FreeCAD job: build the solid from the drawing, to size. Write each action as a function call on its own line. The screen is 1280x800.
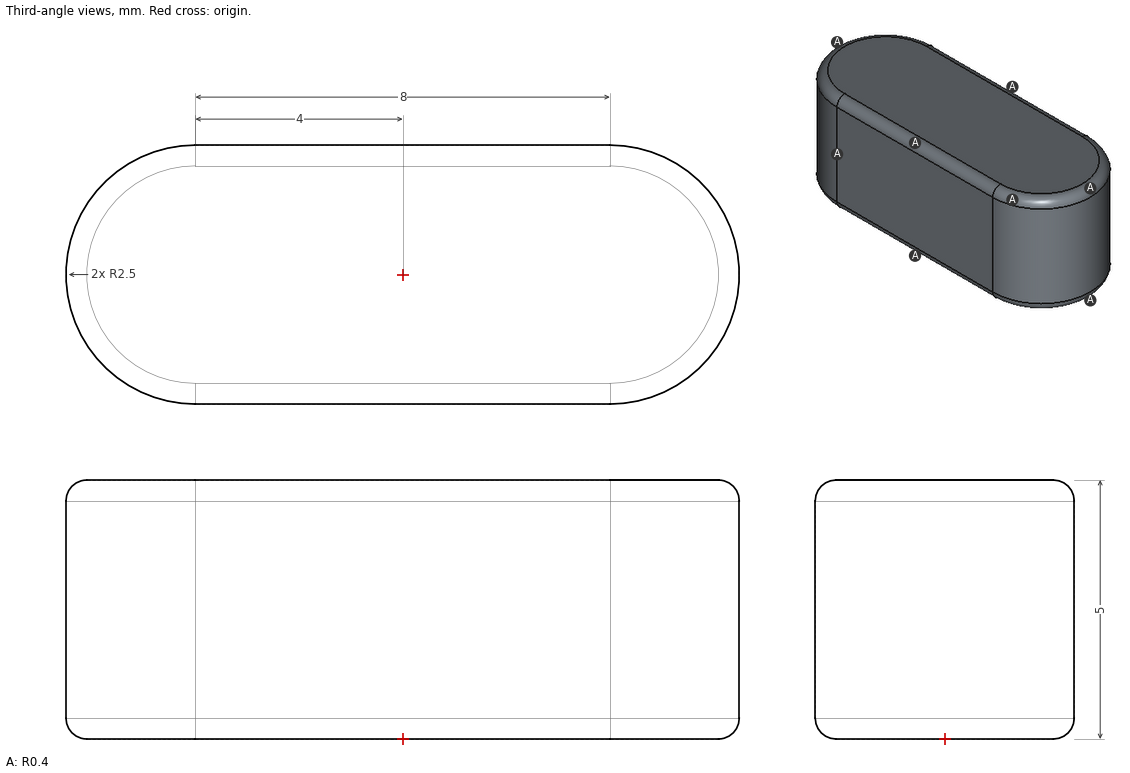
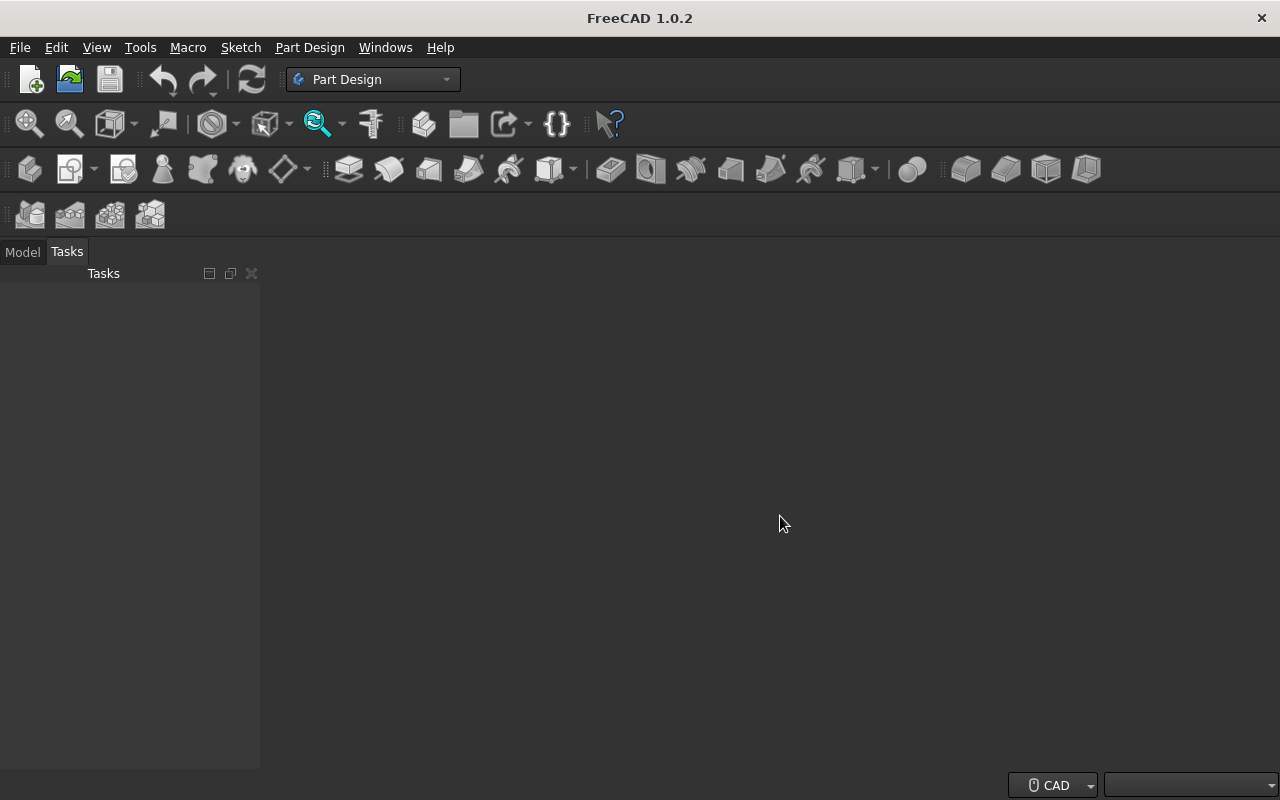
click(30, 80)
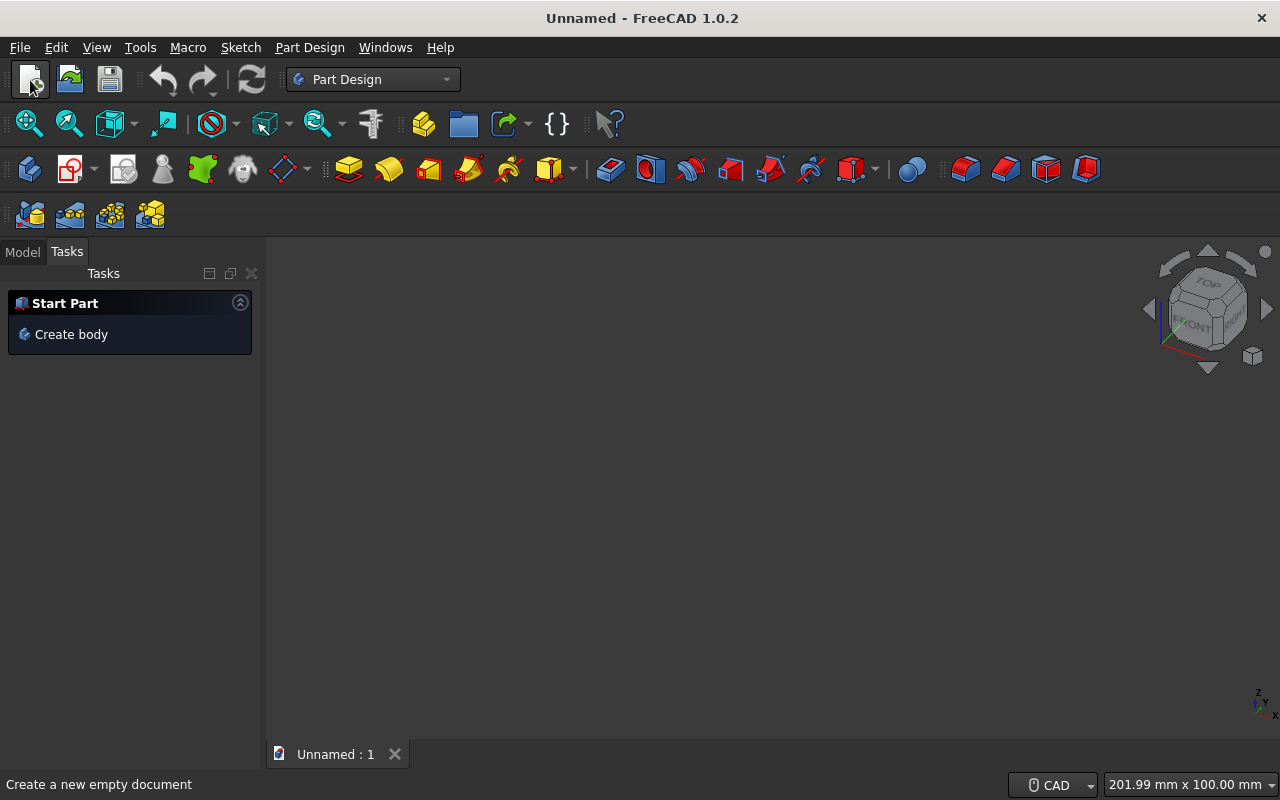
click(70, 170)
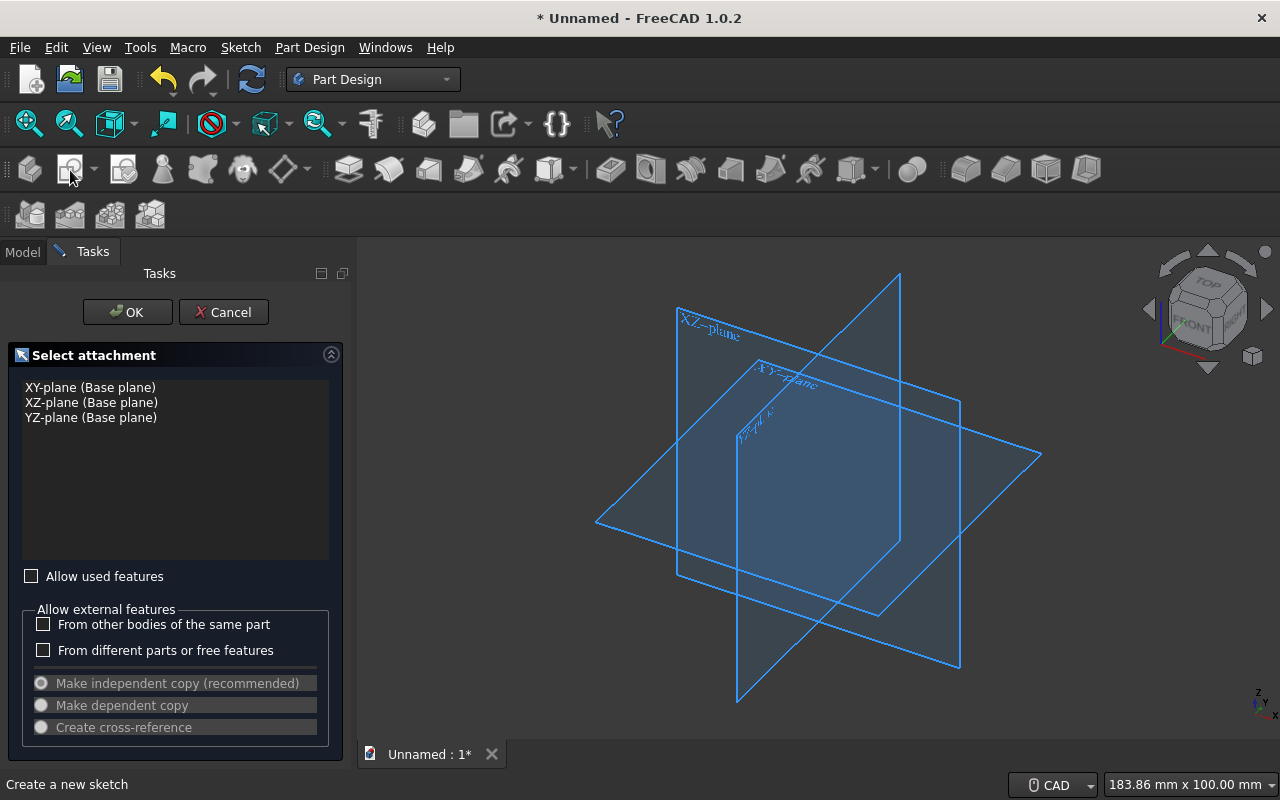
click(82, 388)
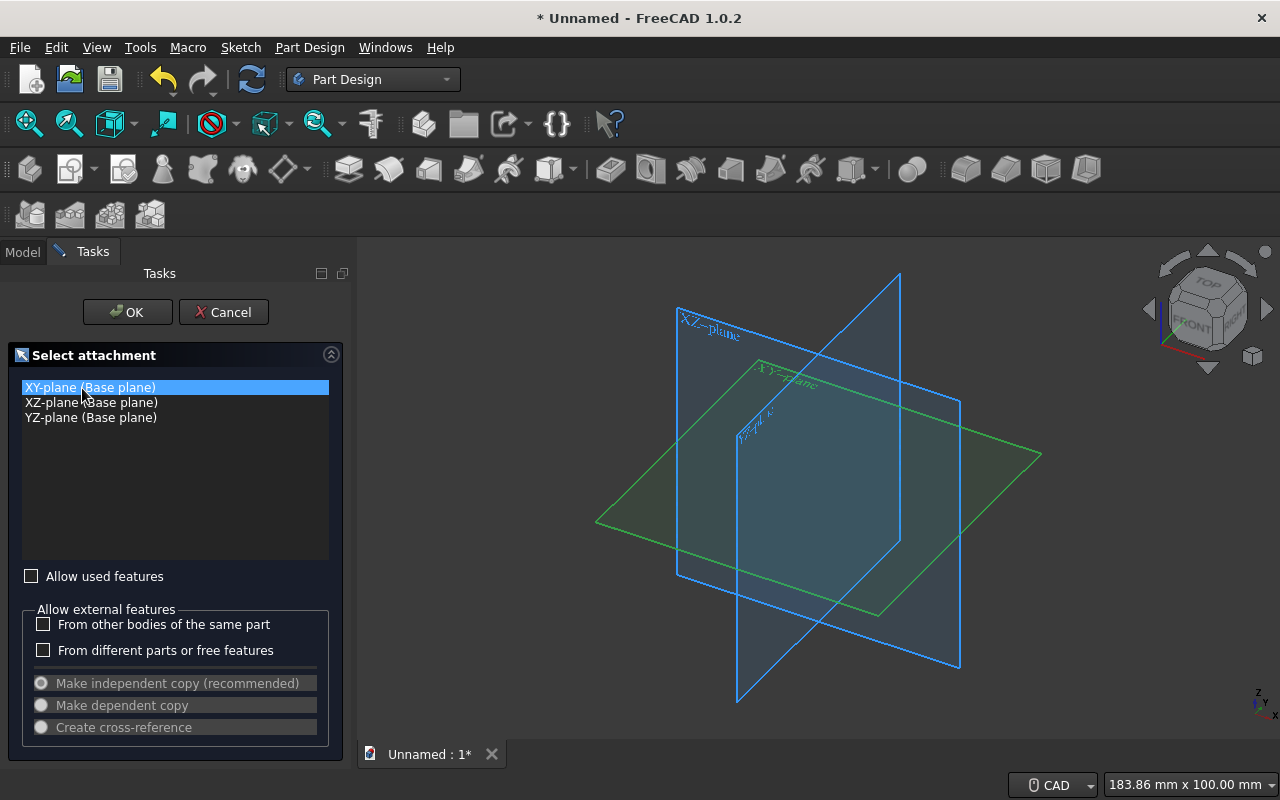
click(128, 312)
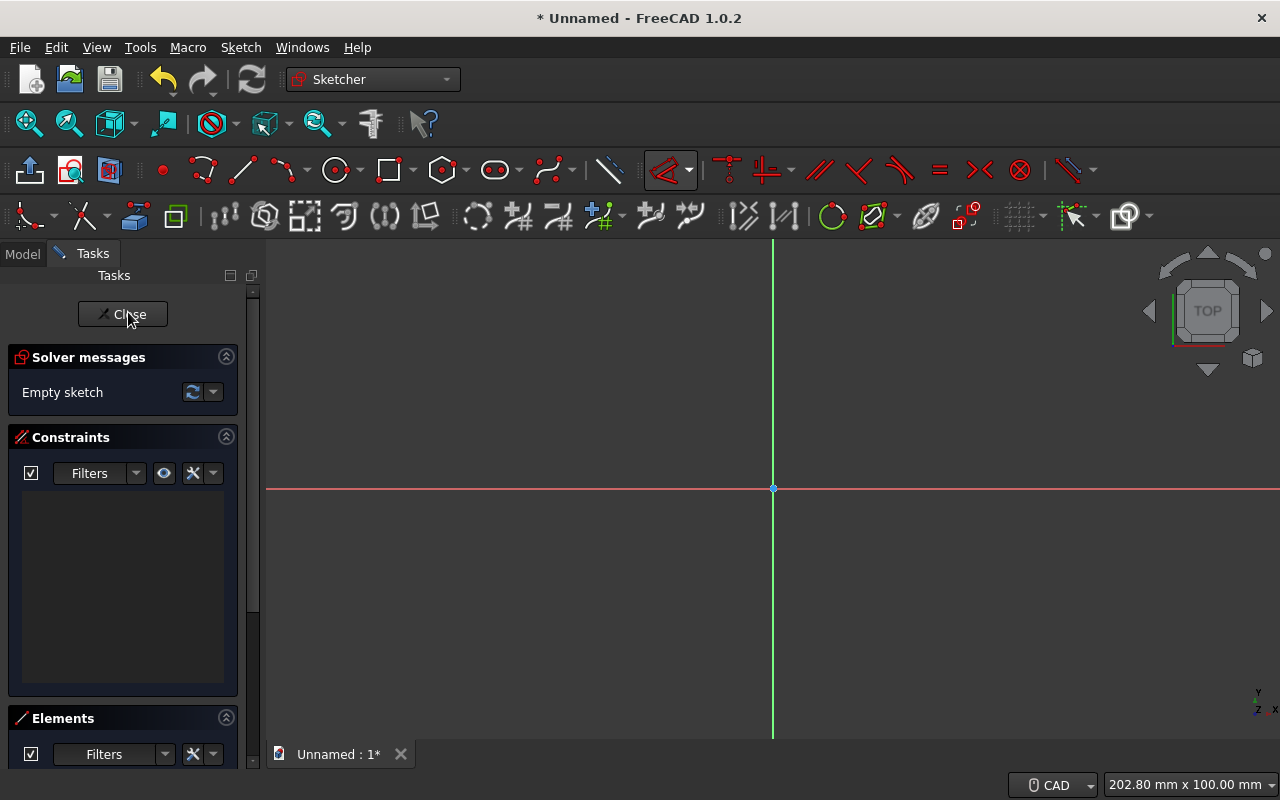
scroll(782, 489, up, 11)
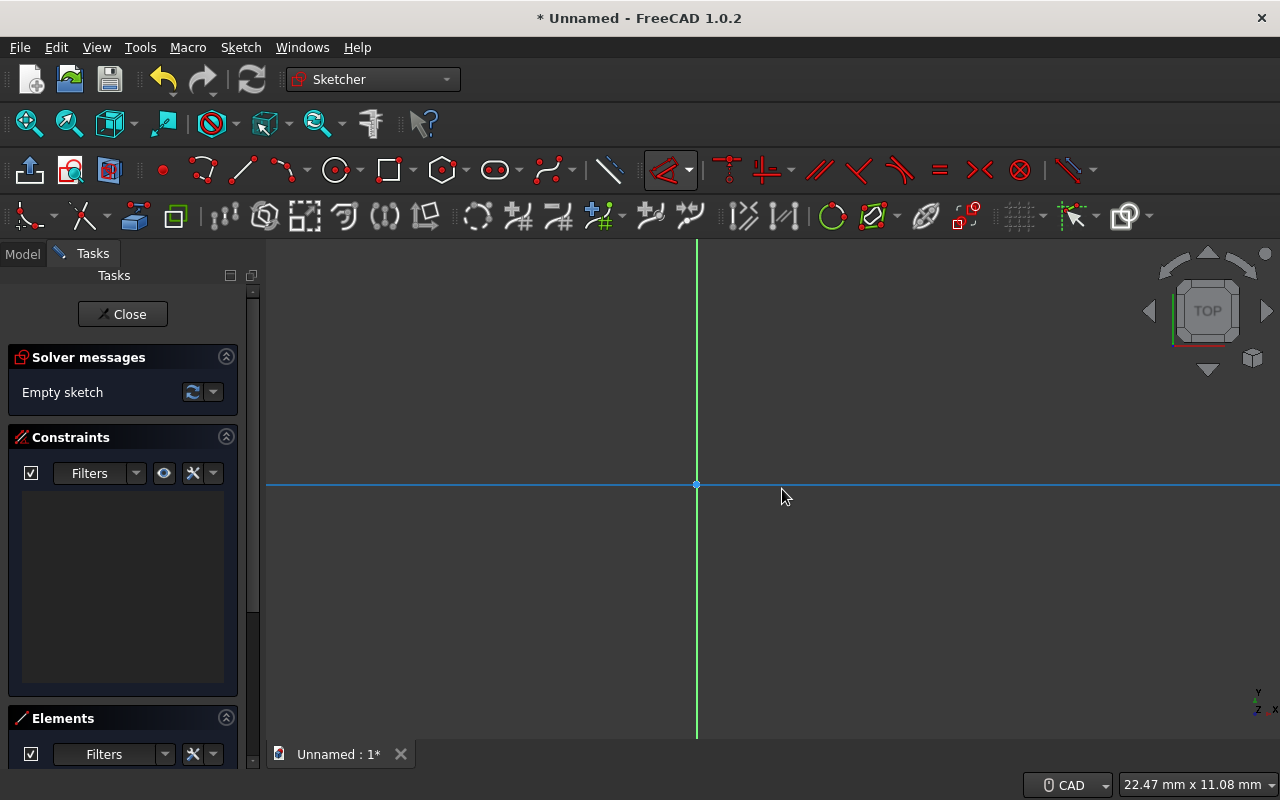
click(496, 170)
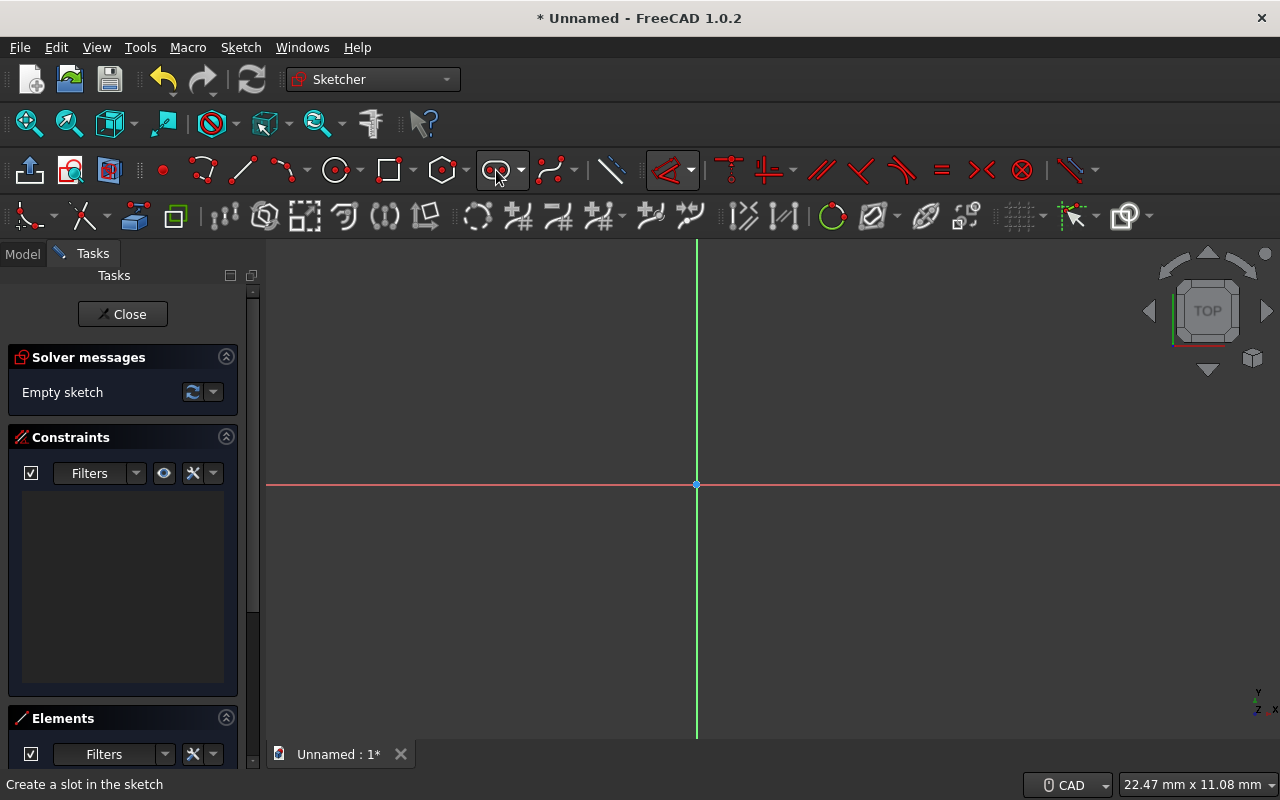
click(516, 485)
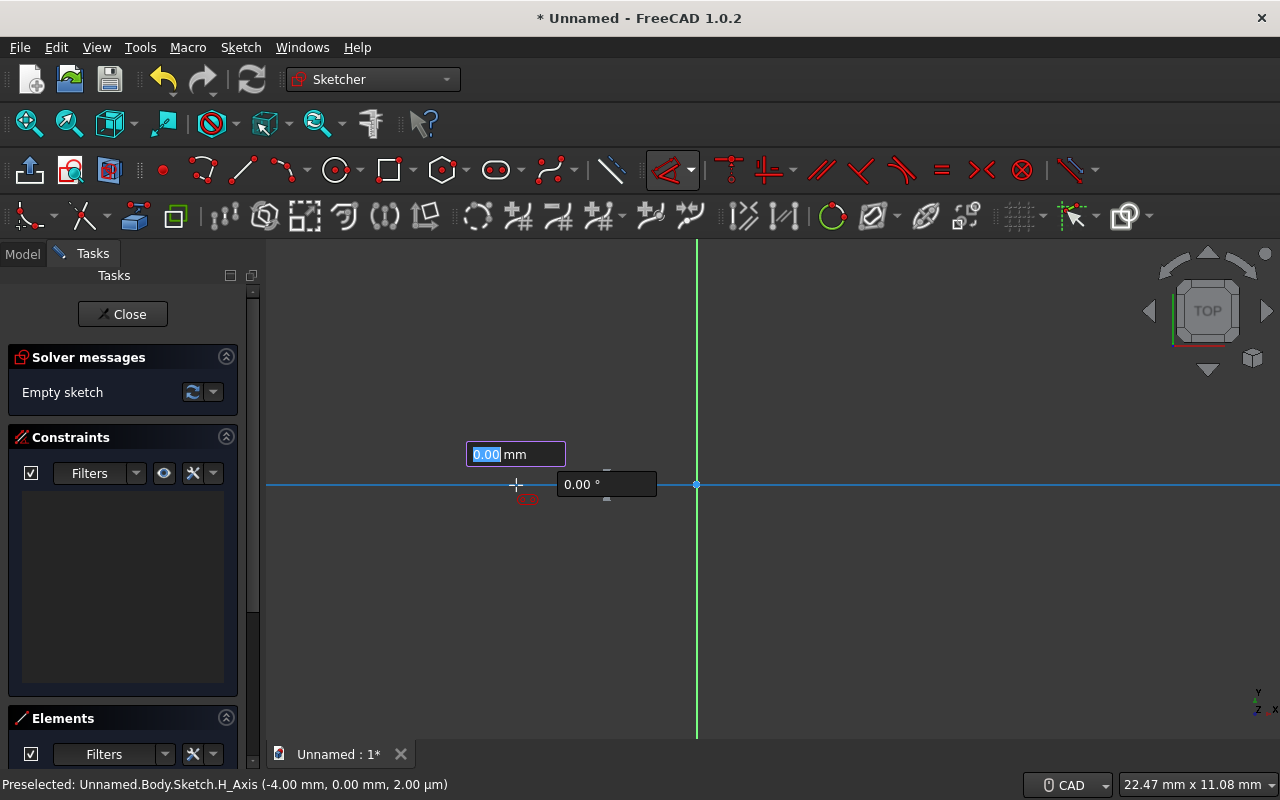
click(877, 476)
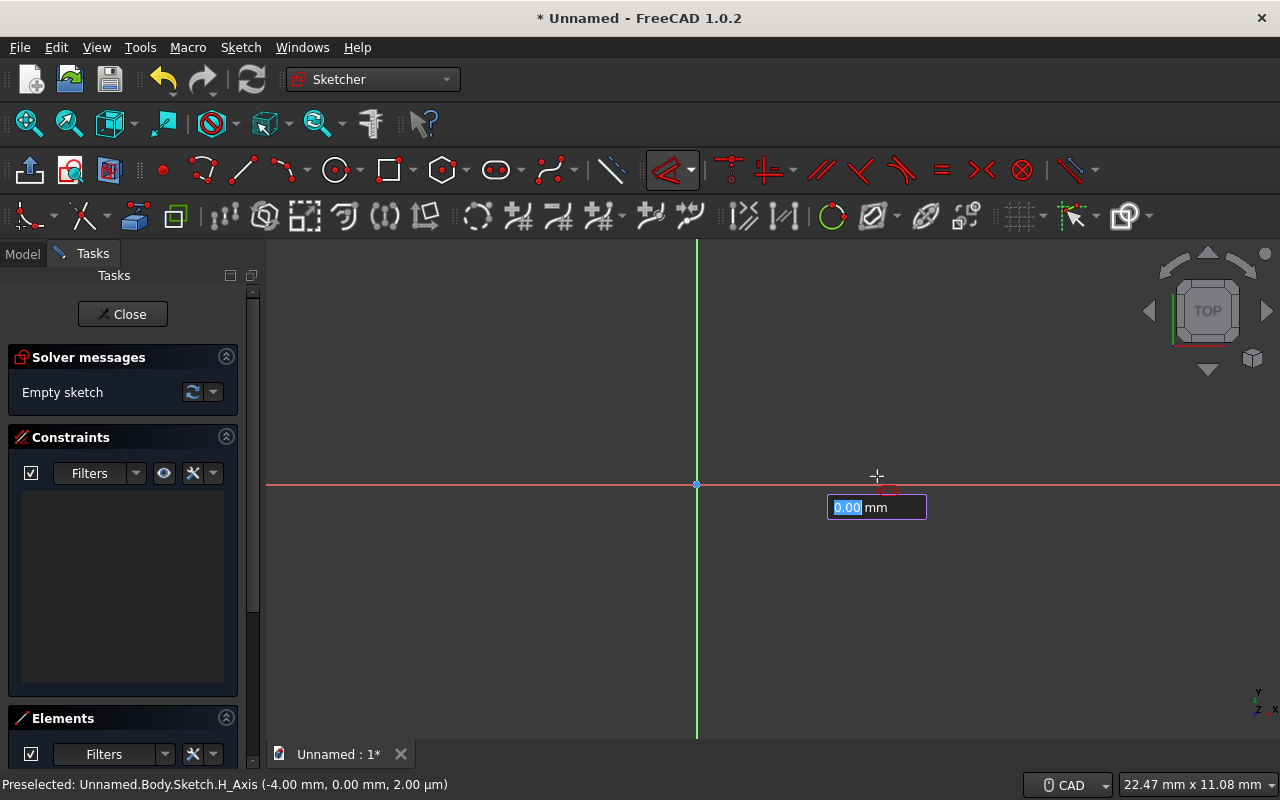
click(751, 372)
key(Escape)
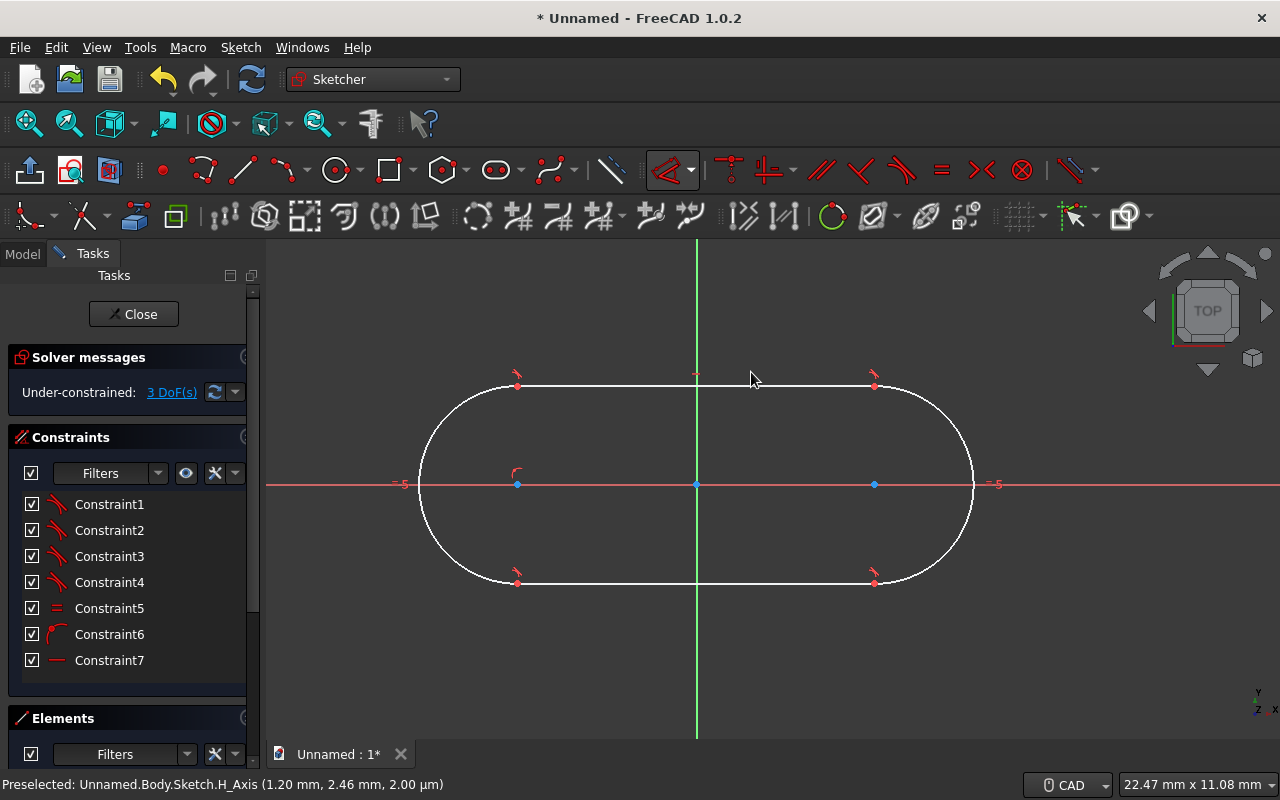
click(438, 427)